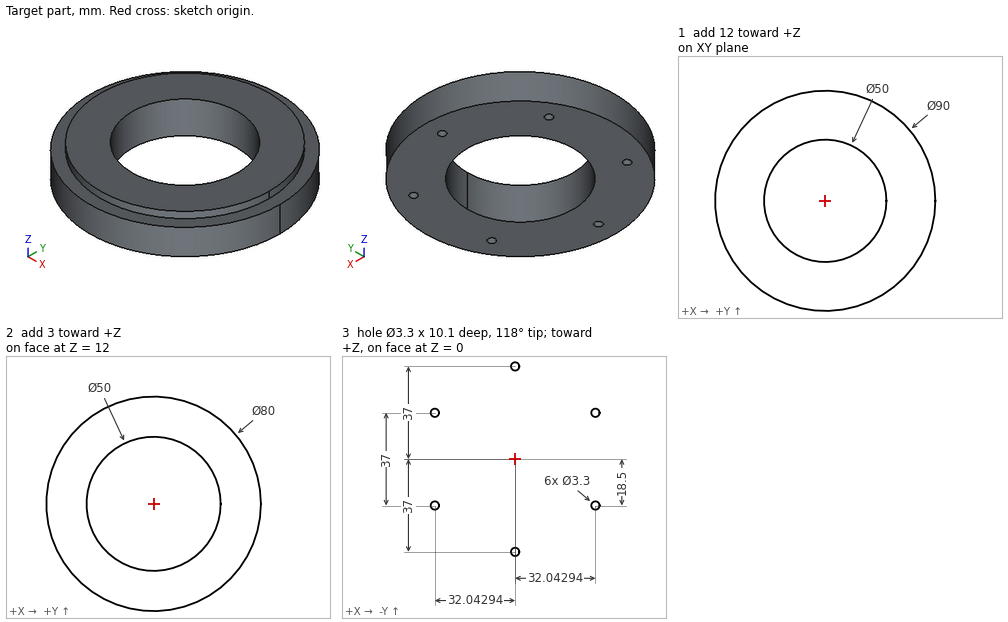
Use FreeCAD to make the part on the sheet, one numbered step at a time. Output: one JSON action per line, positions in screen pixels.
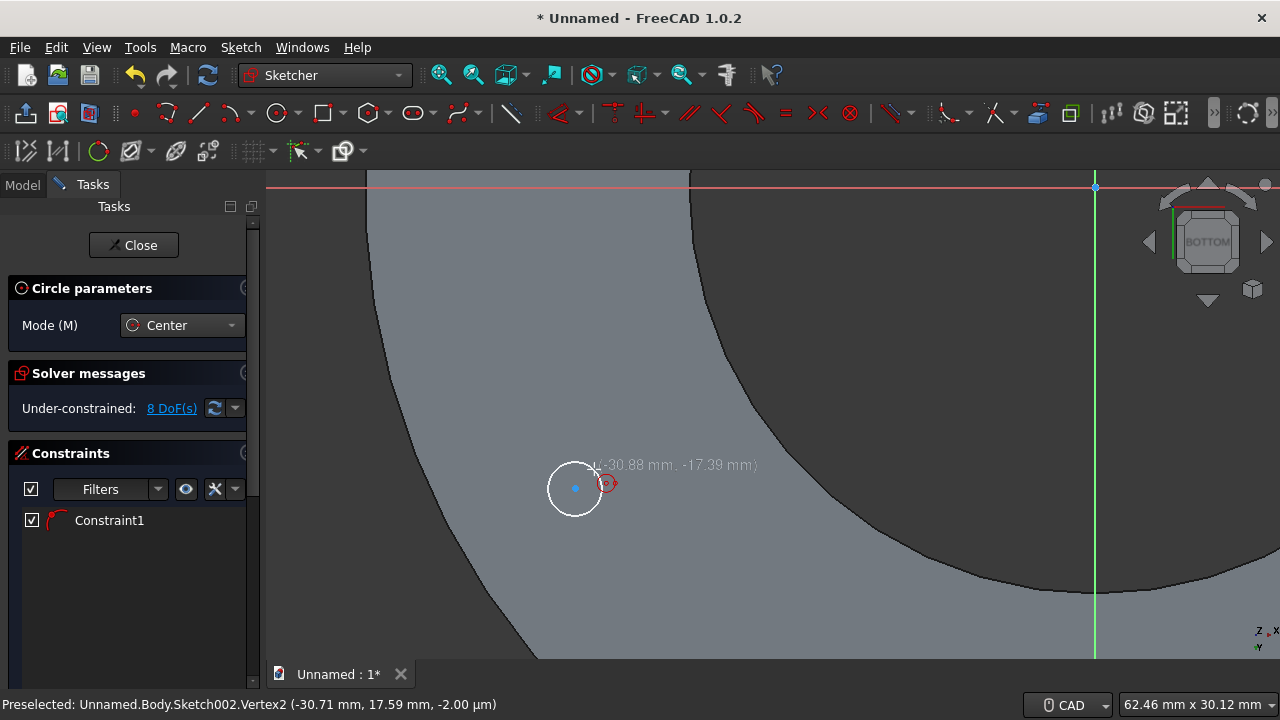
{"action": "scroll", "coordinate": [577, 489], "scroll_direction": "down", "scroll_amount": 7}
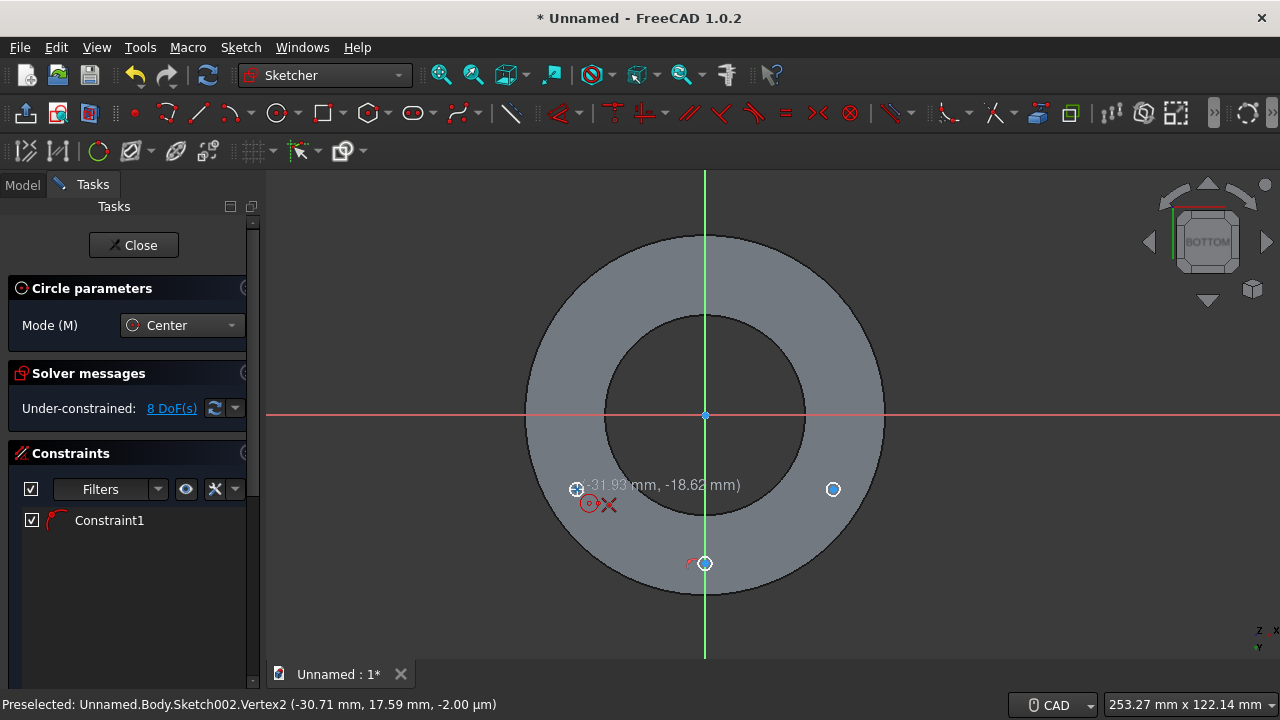
{"action": "scroll", "coordinate": [577, 341], "scroll_direction": "up", "scroll_amount": 7}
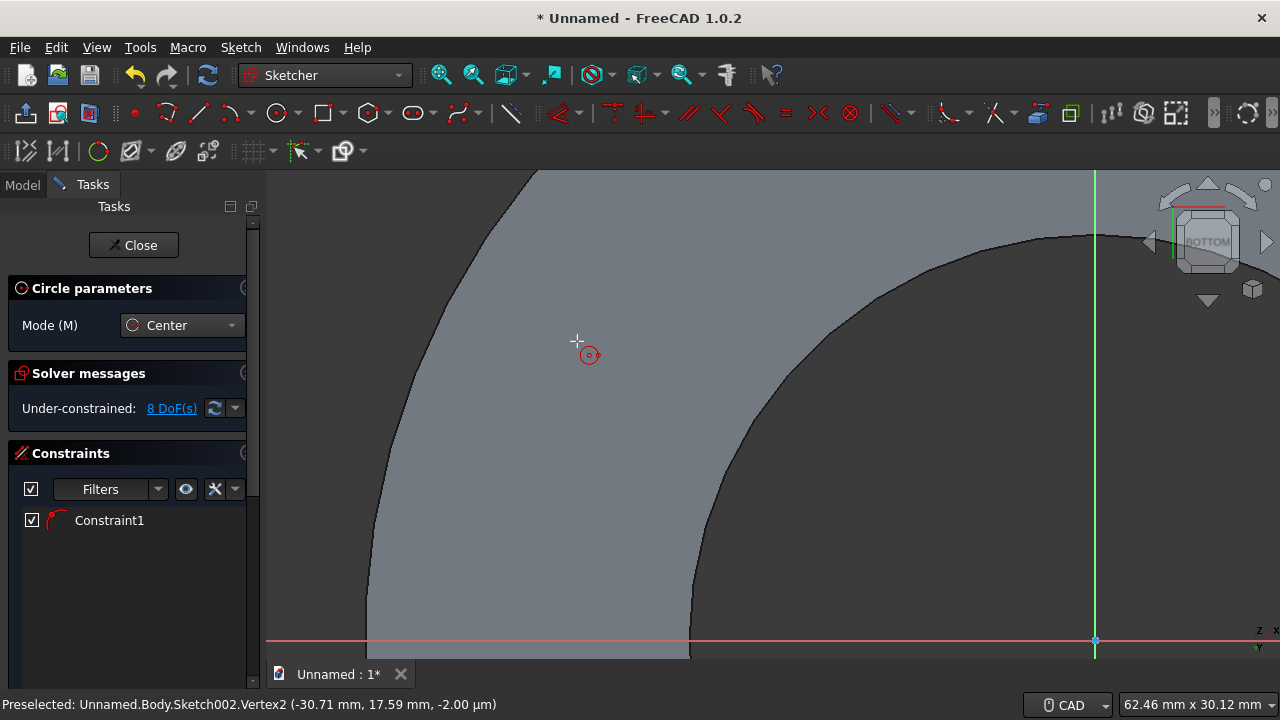
{"action": "left_click", "coordinate": [575, 340]}
{"action": "left_click", "coordinate": [594, 321]}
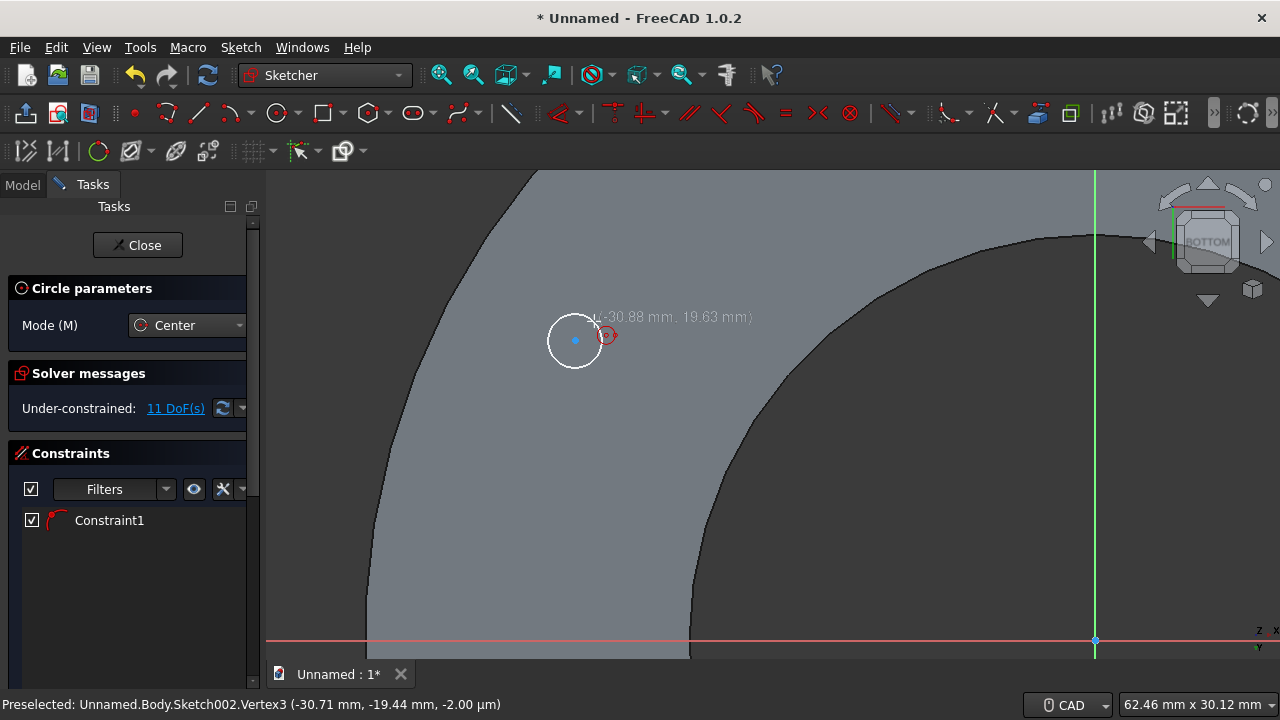
{"action": "scroll", "coordinate": [577, 340], "scroll_direction": "down", "scroll_amount": 7}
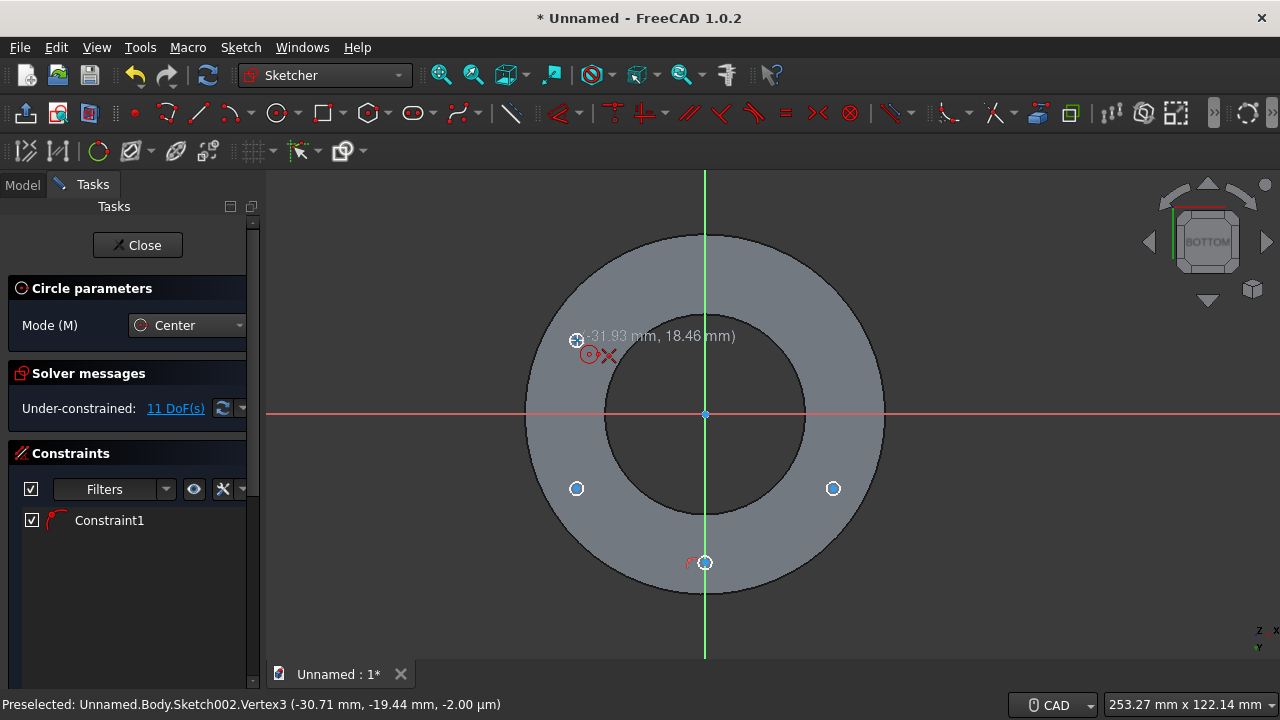
{"action": "scroll", "coordinate": [705, 266], "scroll_direction": "up", "scroll_amount": 7}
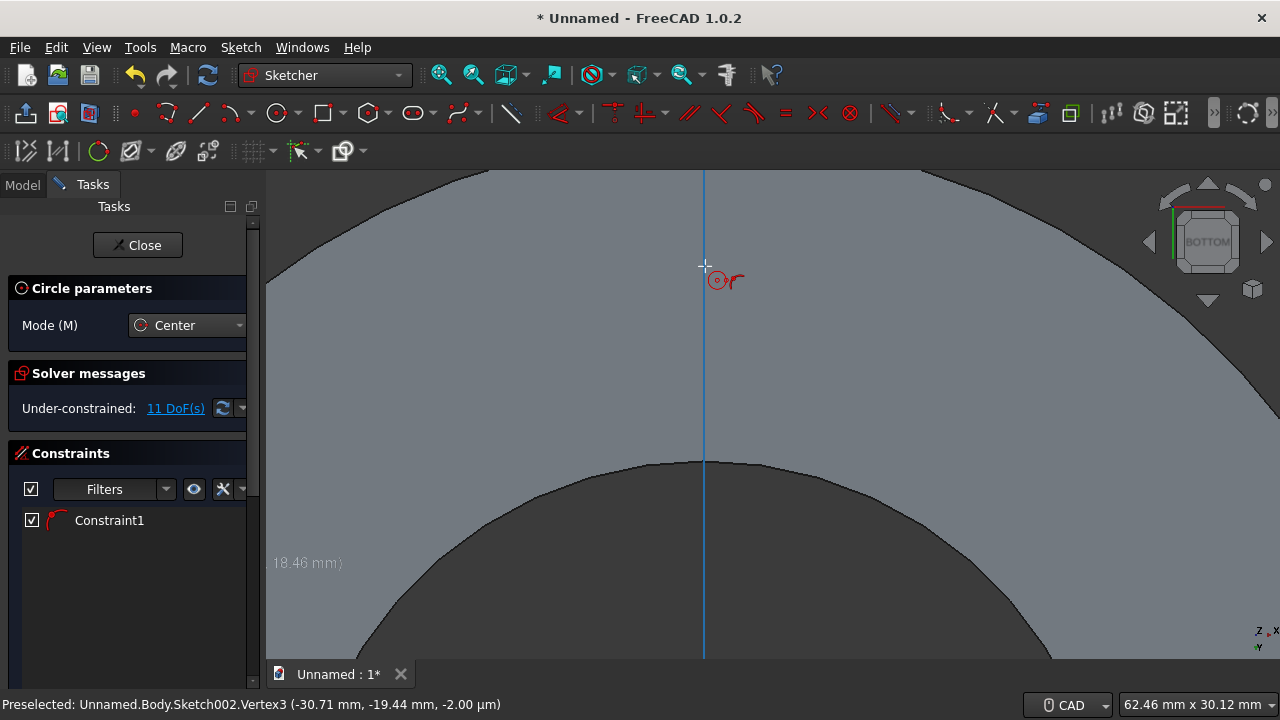
{"action": "left_click", "coordinate": [704, 267]}
{"action": "left_click", "coordinate": [723, 248]}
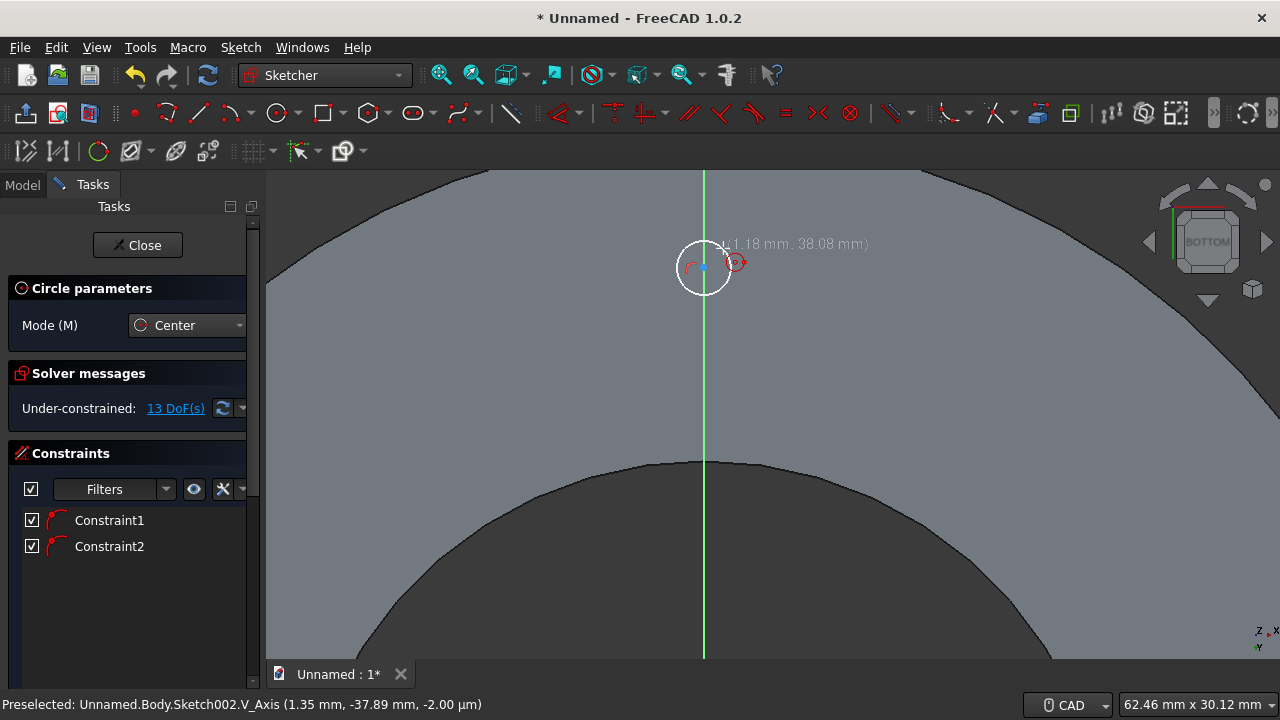
{"action": "scroll", "coordinate": [705, 266], "scroll_direction": "down", "scroll_amount": 7}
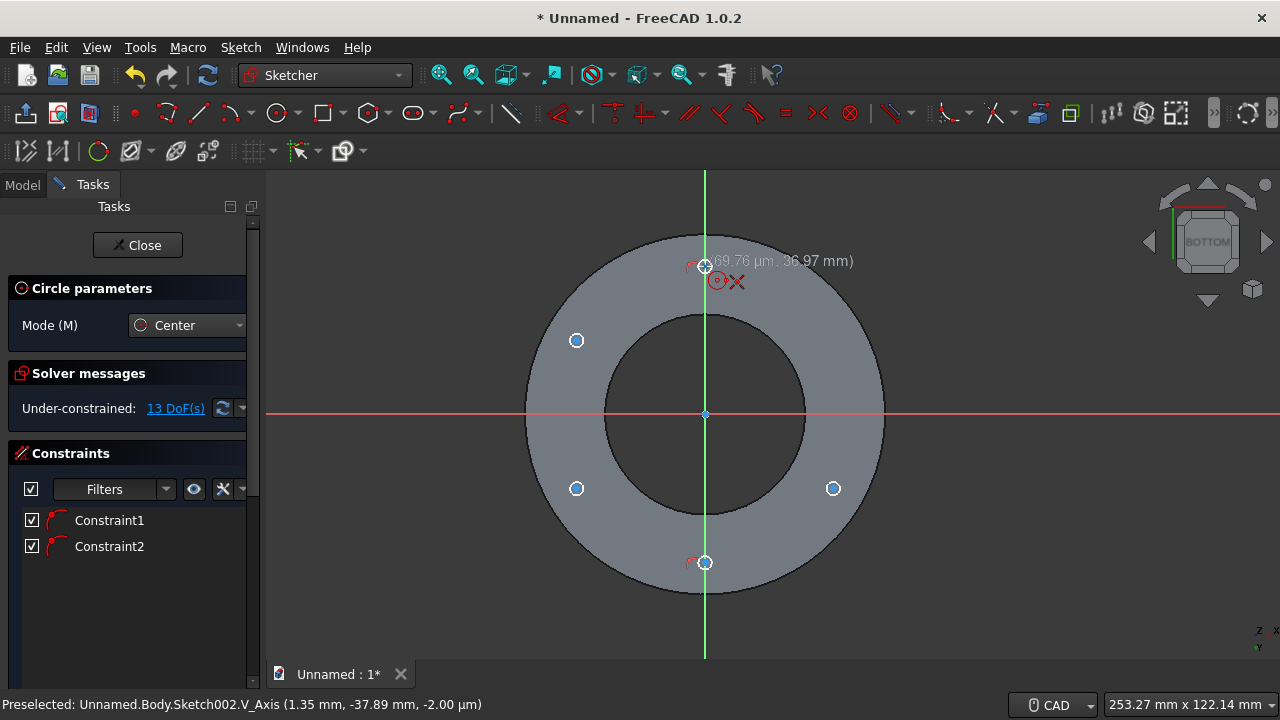
{"action": "scroll", "coordinate": [833, 340], "scroll_direction": "up", "scroll_amount": 7}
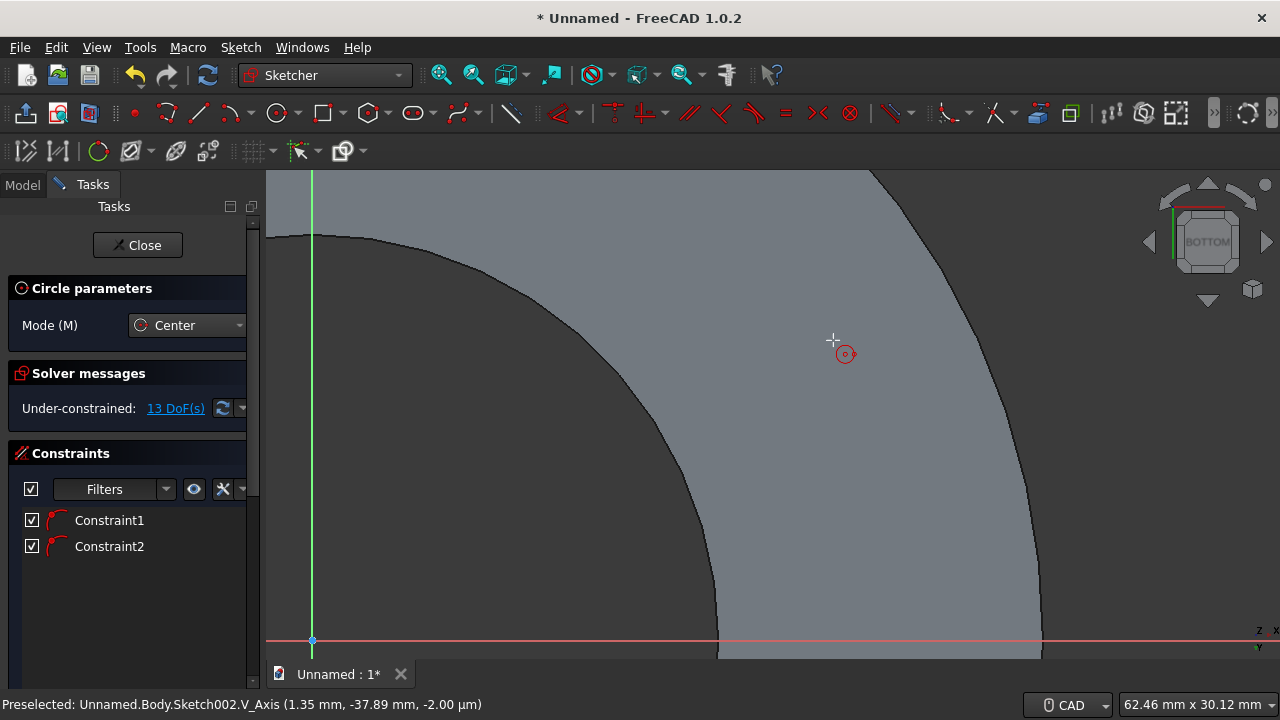
{"action": "left_click", "coordinate": [833, 340]}
{"action": "left_click", "coordinate": [852, 321]}
{"action": "key", "text": "Escape"}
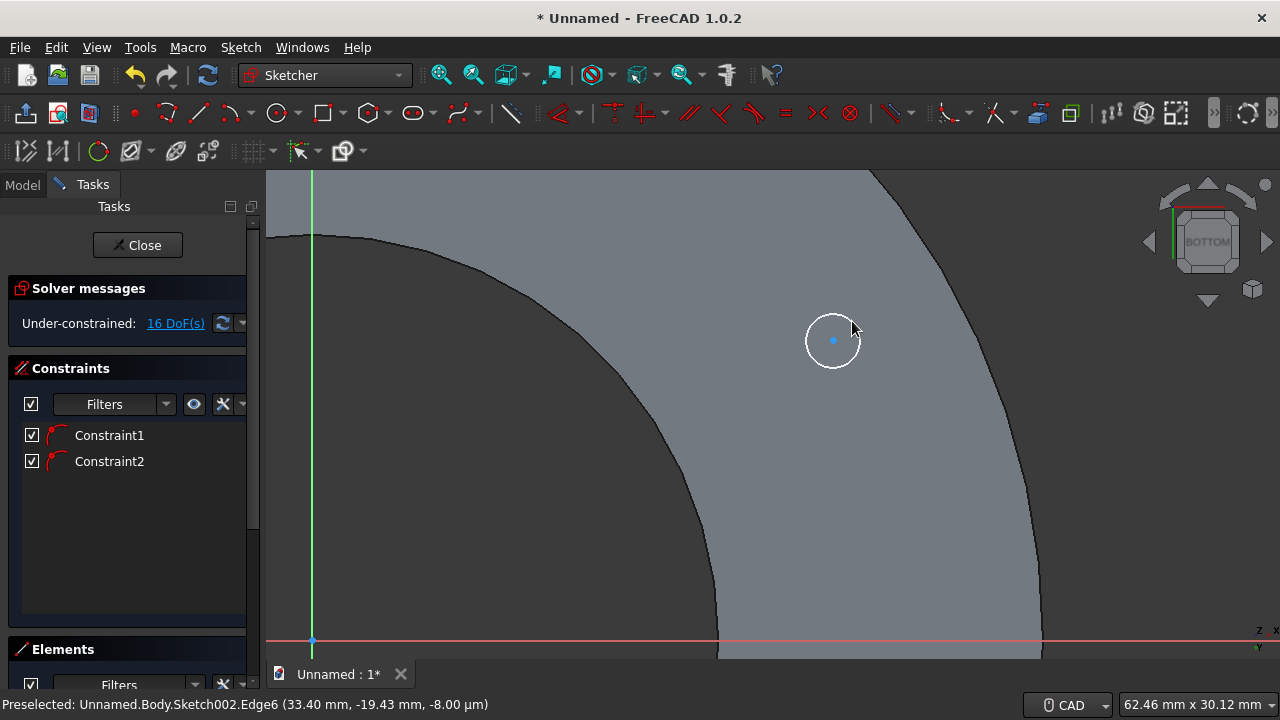
{"action": "scroll", "coordinate": [833, 340], "scroll_direction": "down", "scroll_amount": 7}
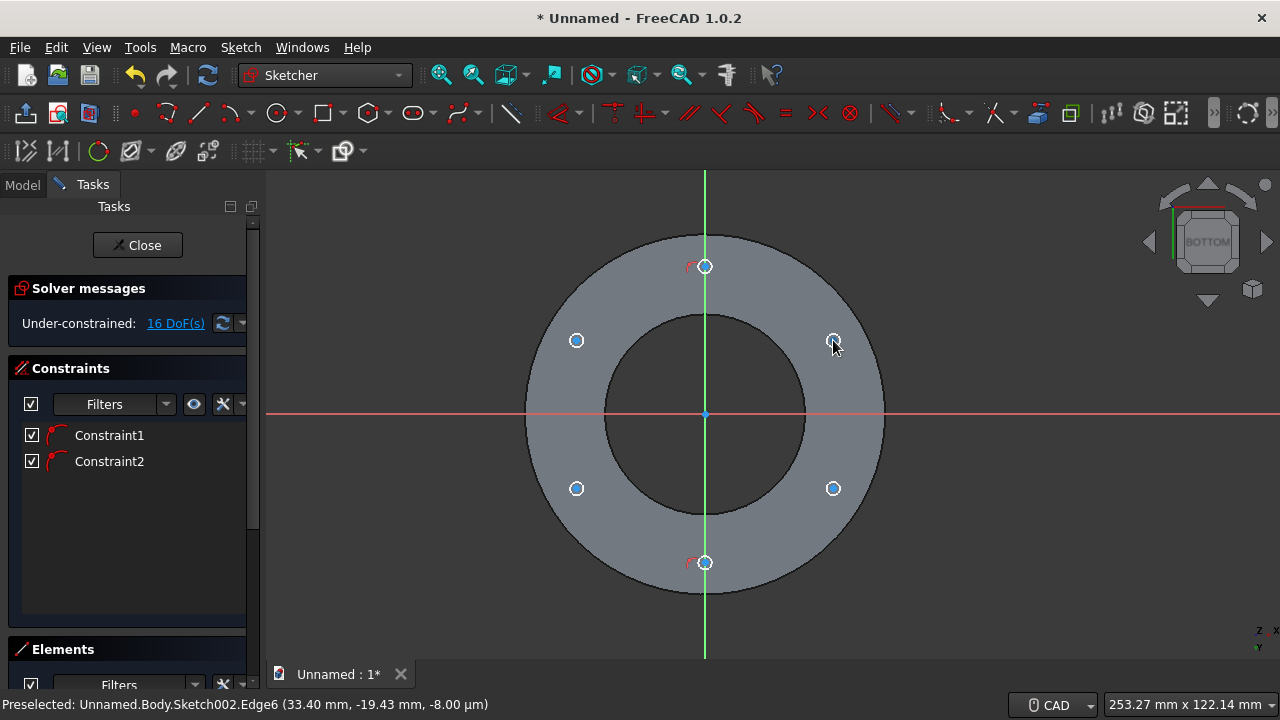
{"action": "scroll", "coordinate": [838, 484], "scroll_direction": "up", "scroll_amount": 4}